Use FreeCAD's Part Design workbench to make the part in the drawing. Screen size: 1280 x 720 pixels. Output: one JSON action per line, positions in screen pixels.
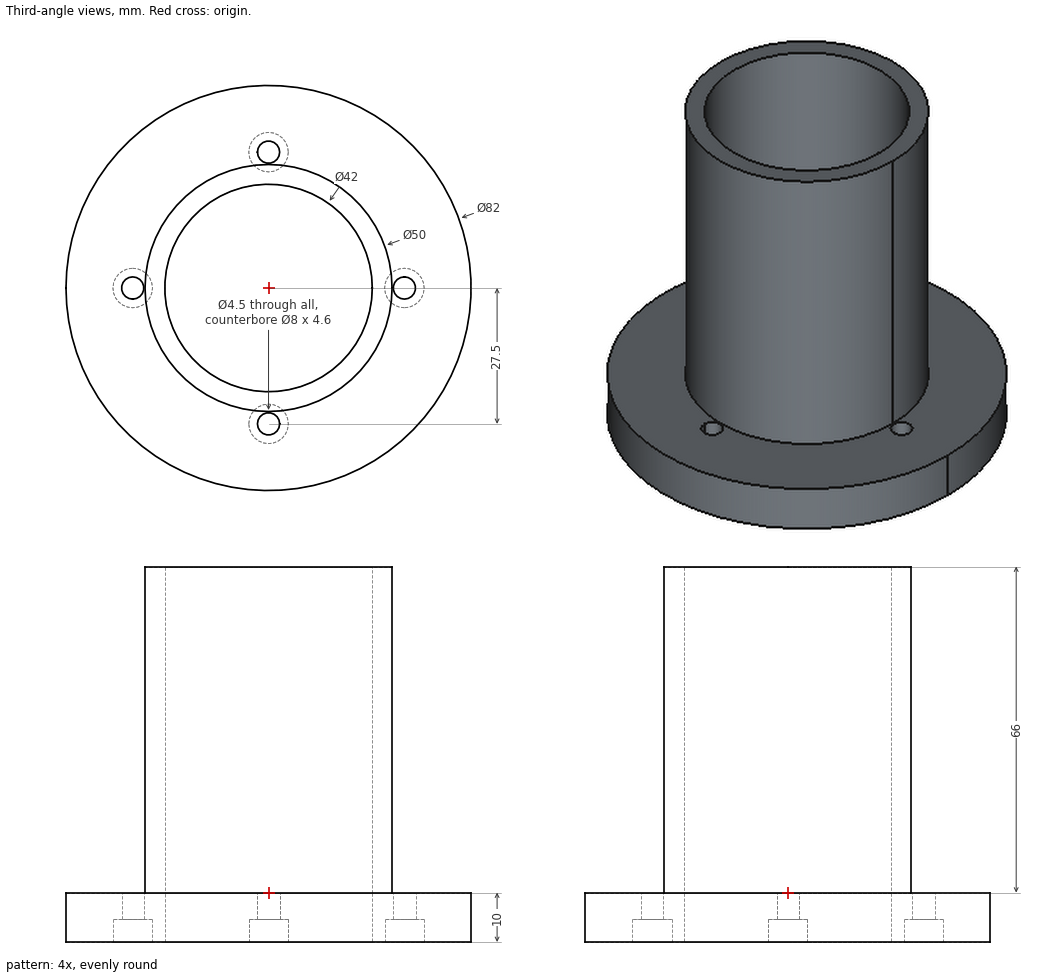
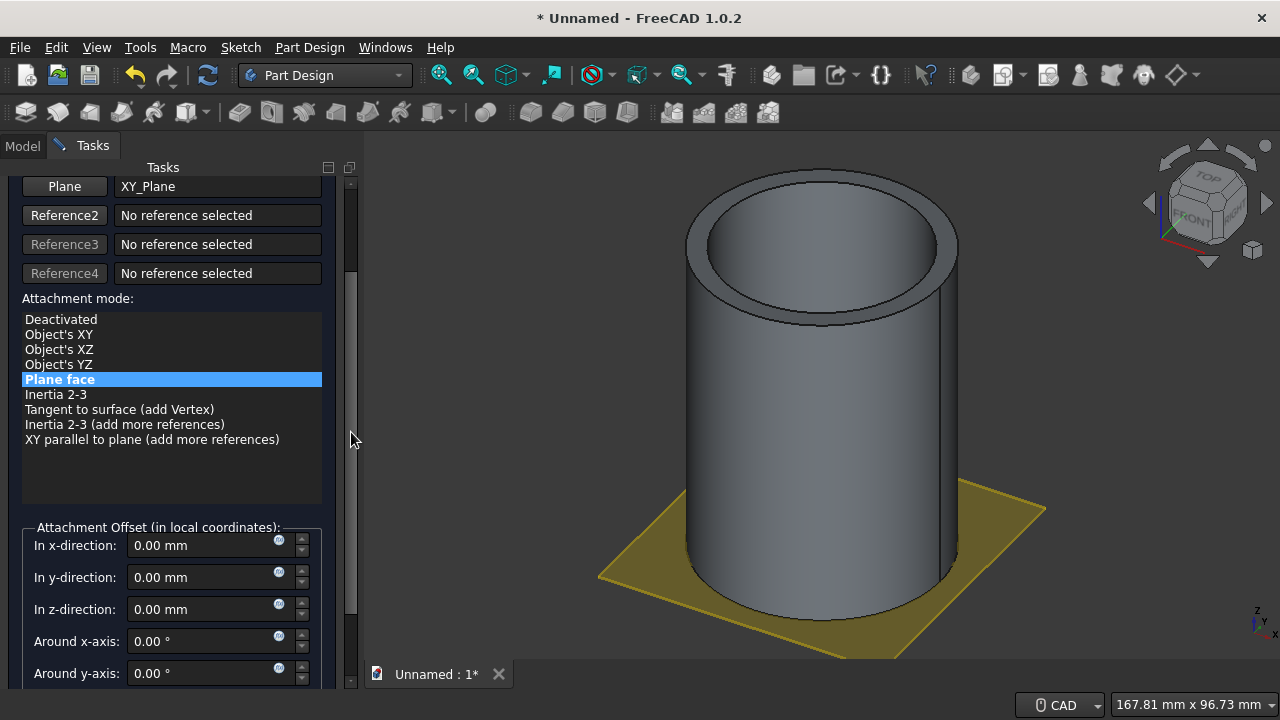
{"action": "triple_click", "coordinate": [210, 609]}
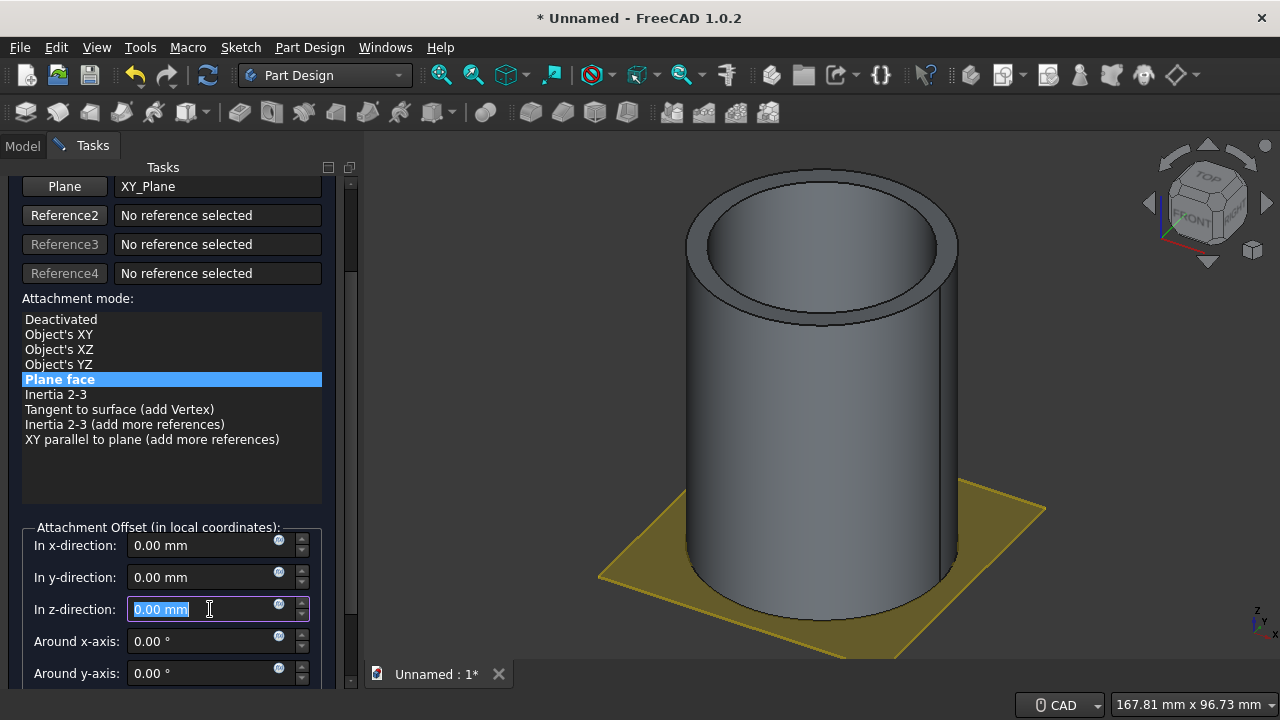
{"action": "type", "text": "-10"}
{"action": "key", "text": "Tab"}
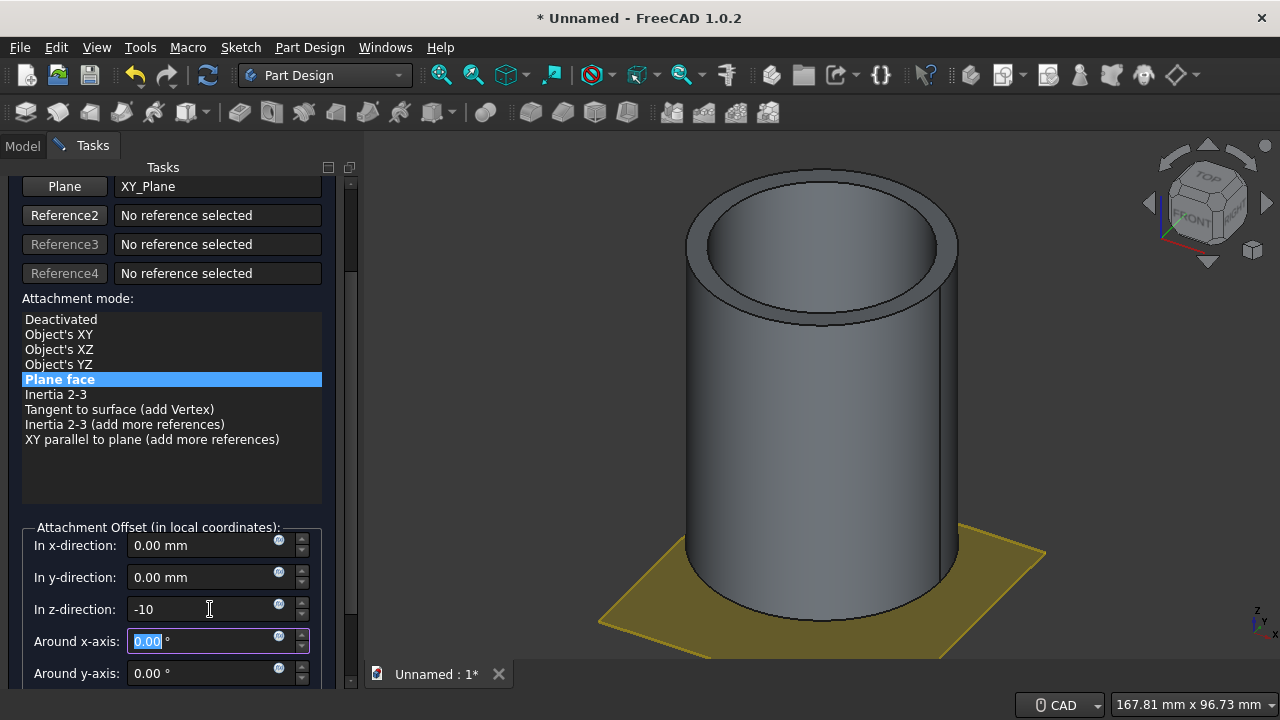
{"action": "scroll", "coordinate": [351, 432], "scroll_direction": "up", "scroll_amount": 3}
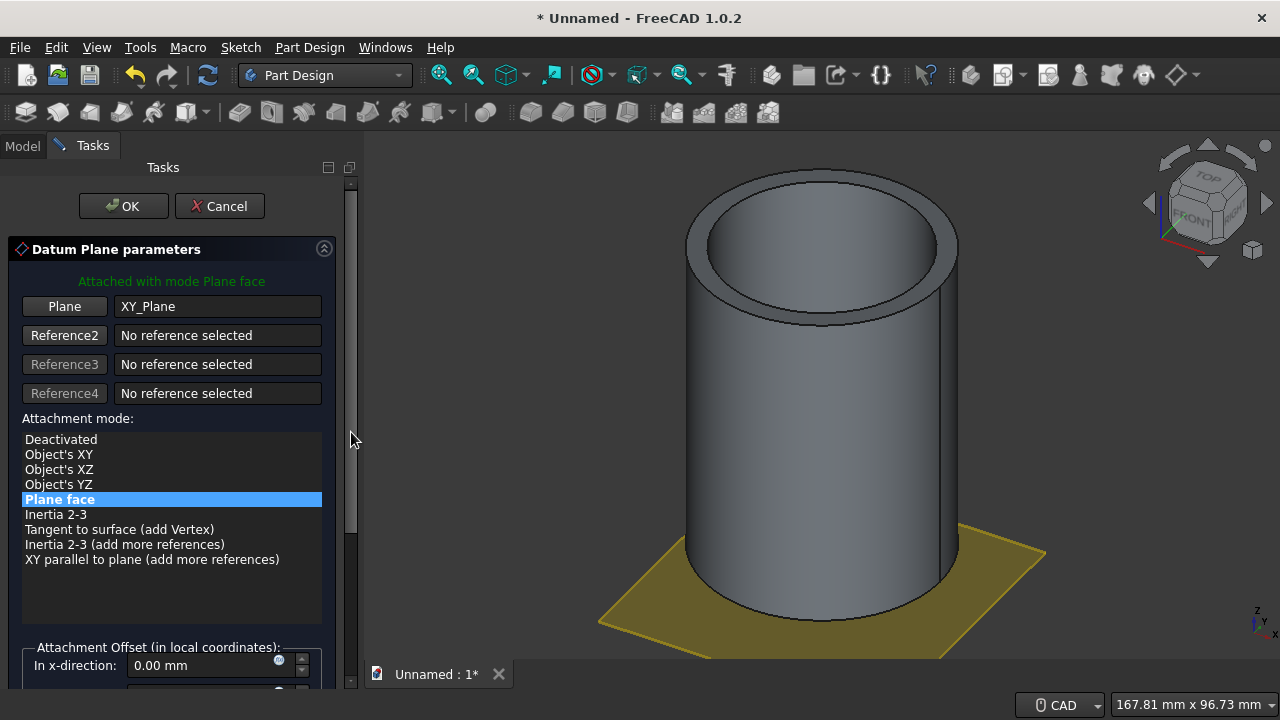
{"action": "left_click", "coordinate": [124, 206]}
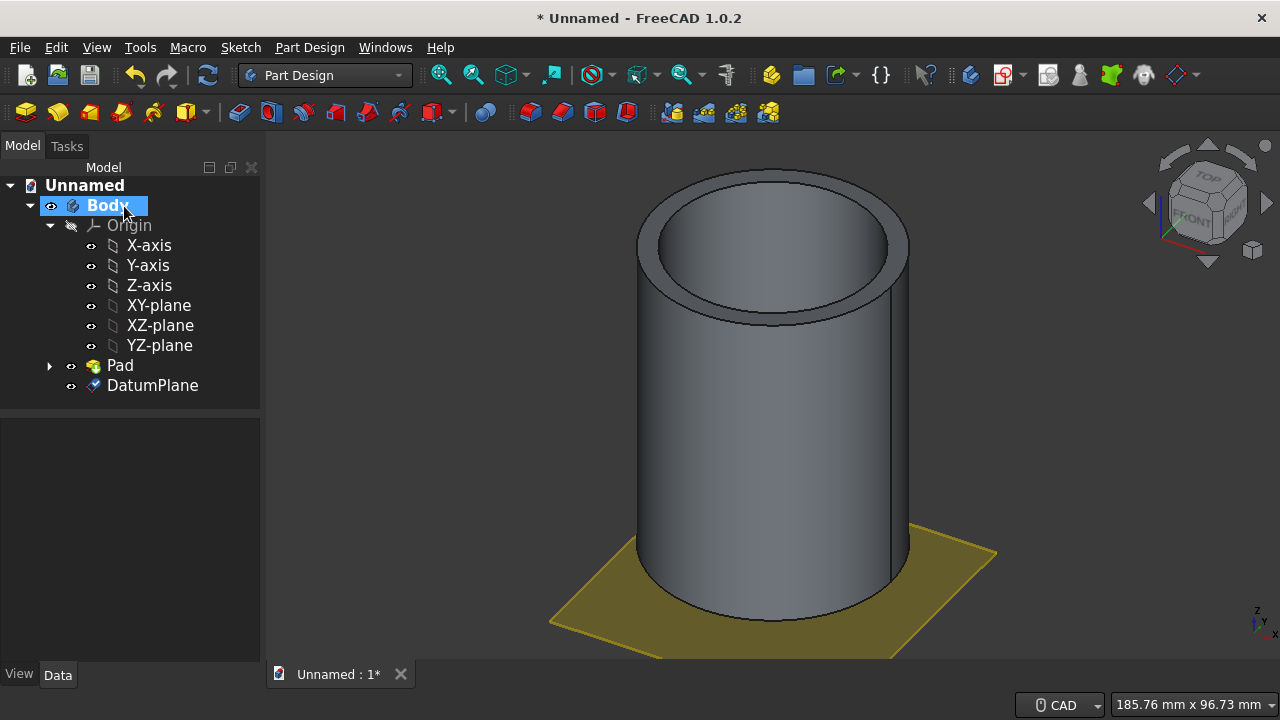
{"action": "left_click", "coordinate": [116, 386]}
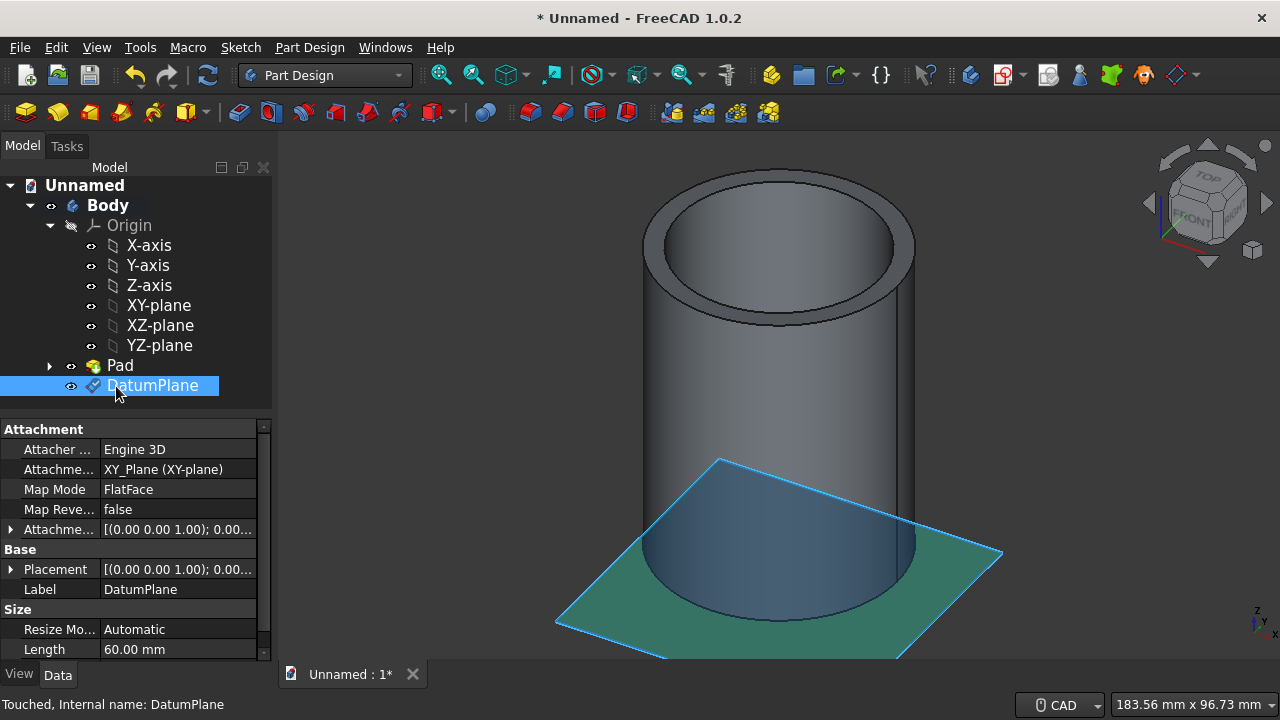
{"action": "left_click", "coordinate": [1004, 76]}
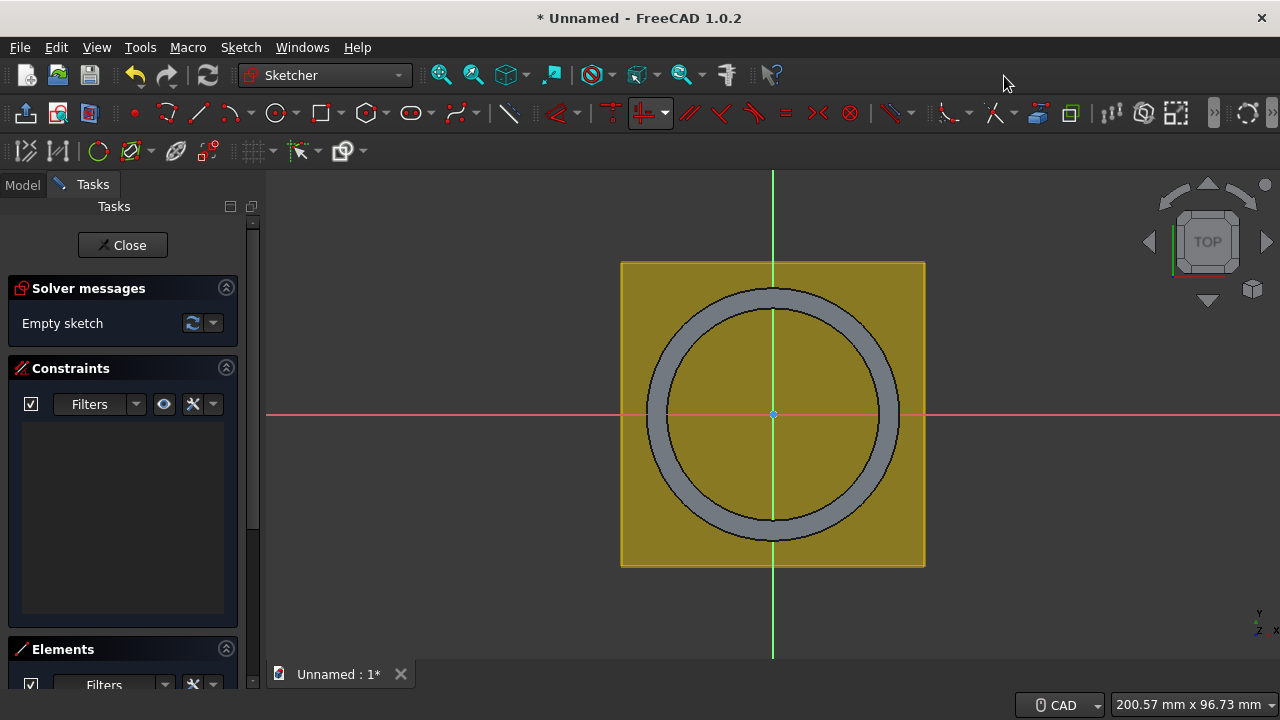
{"action": "left_click", "coordinate": [90, 114]}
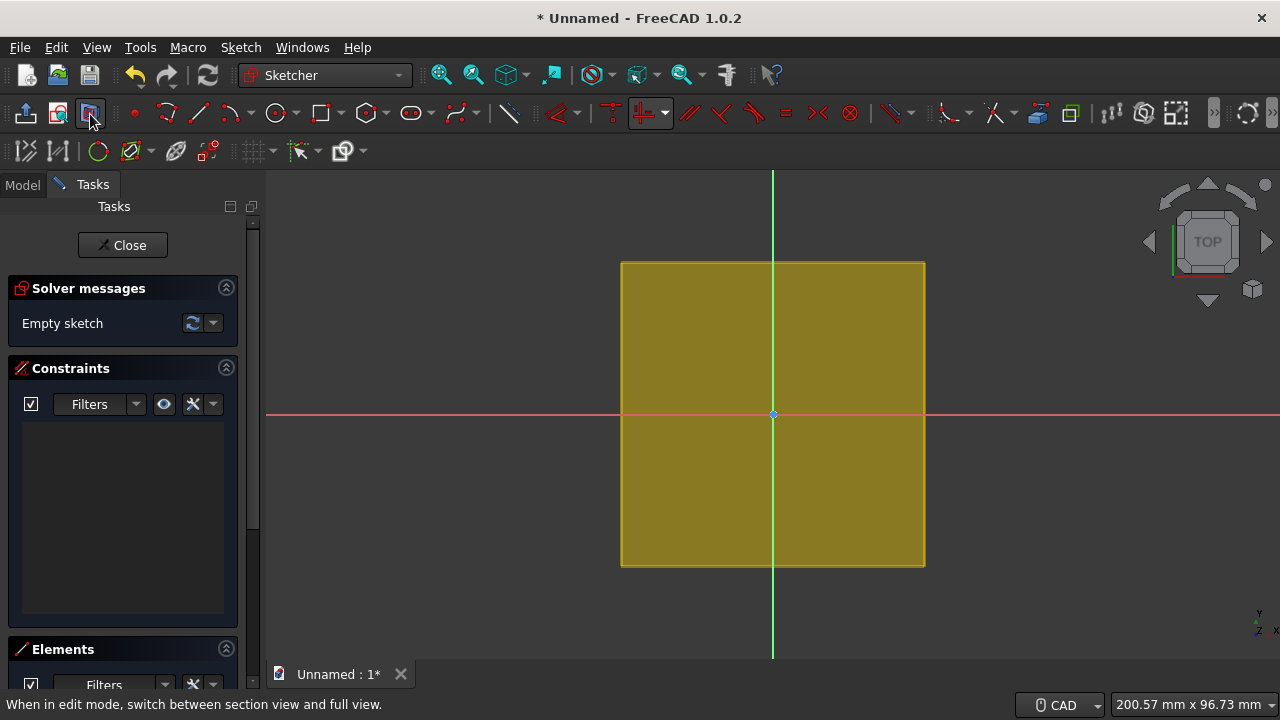
{"action": "scroll", "coordinate": [565, 414], "scroll_direction": "down", "scroll_amount": 2}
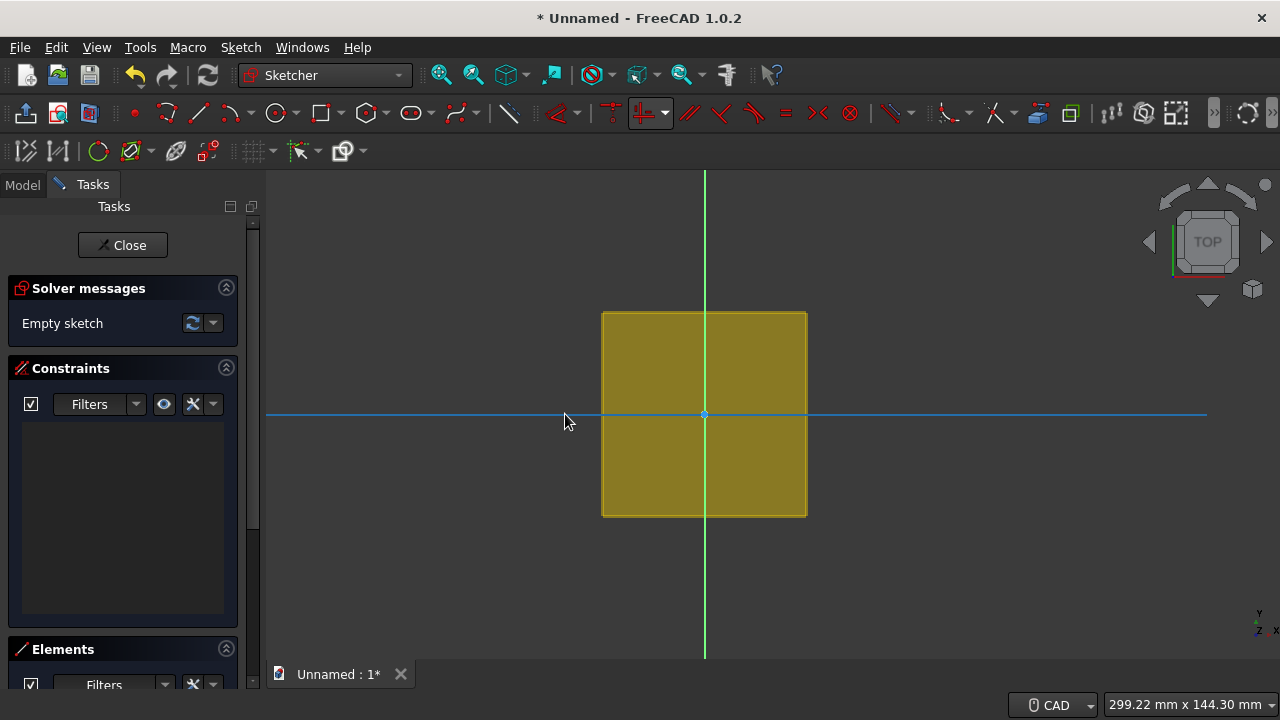
{"action": "left_click", "coordinate": [276, 114]}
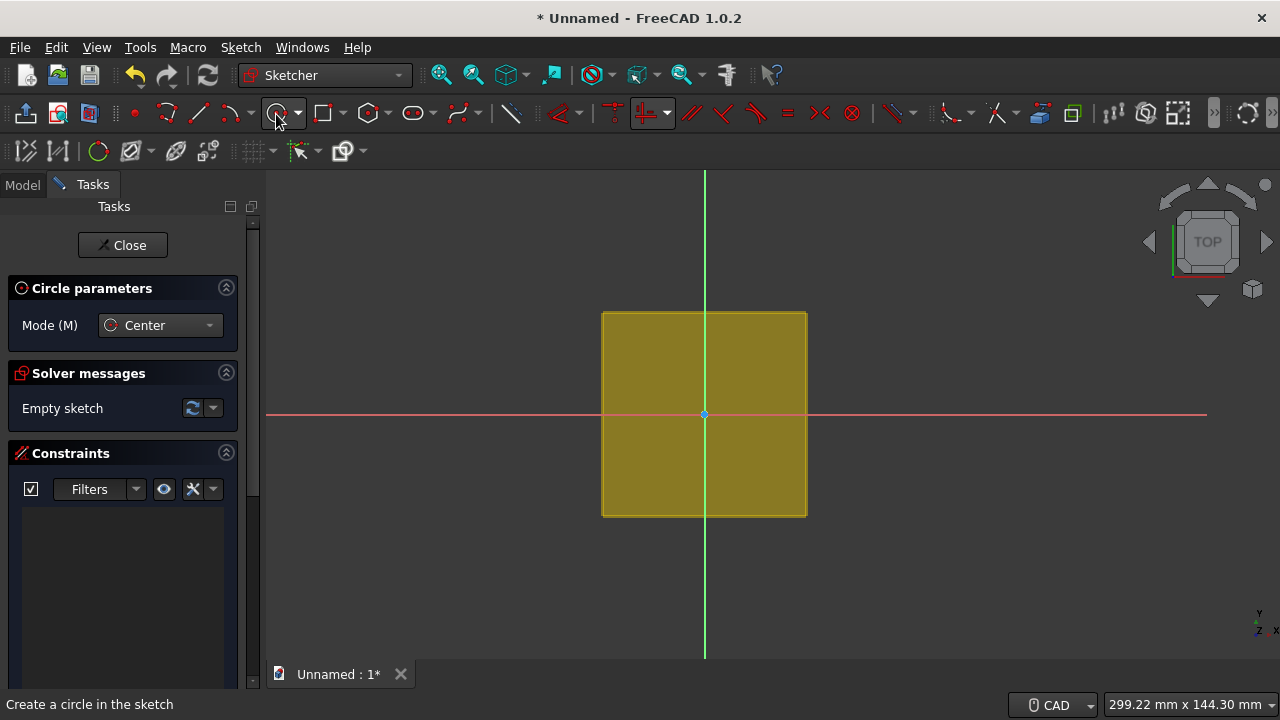
{"action": "left_click", "coordinate": [705, 414]}
{"action": "left_click", "coordinate": [803, 316]}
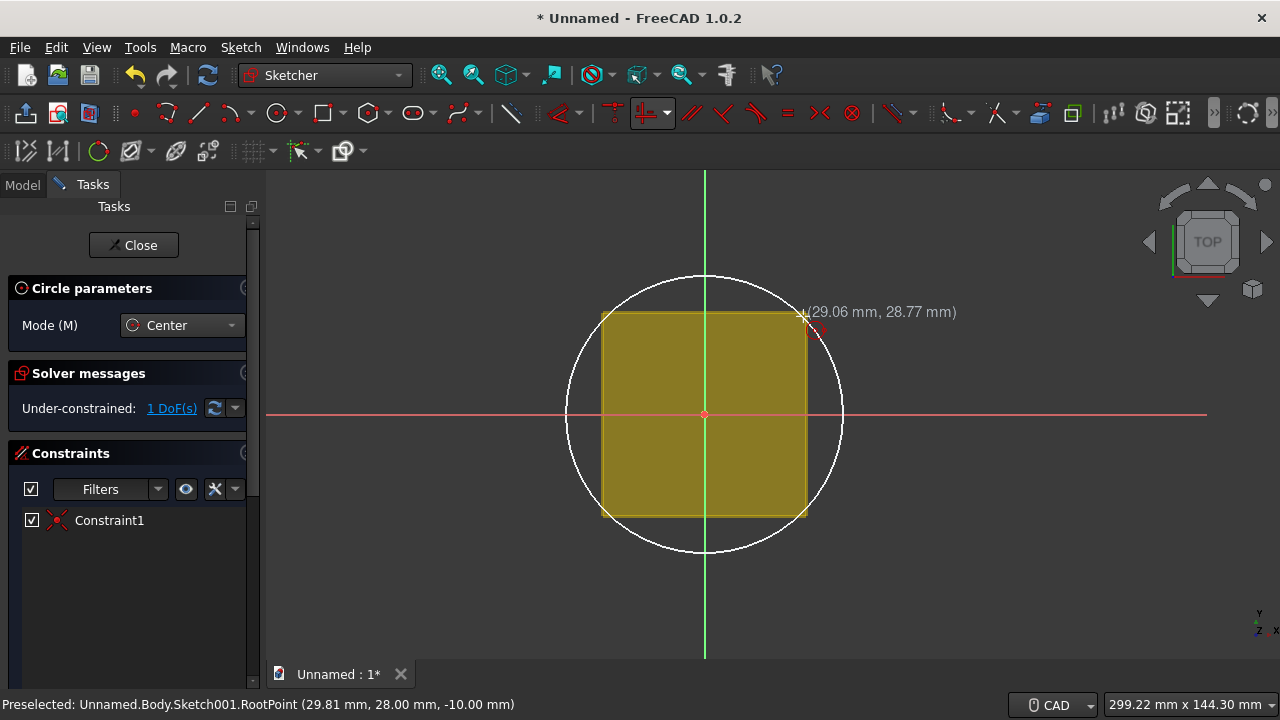
{"action": "left_click", "coordinate": [705, 414]}
{"action": "left_click", "coordinate": [755, 364]}
{"action": "key", "text": "Escape"}